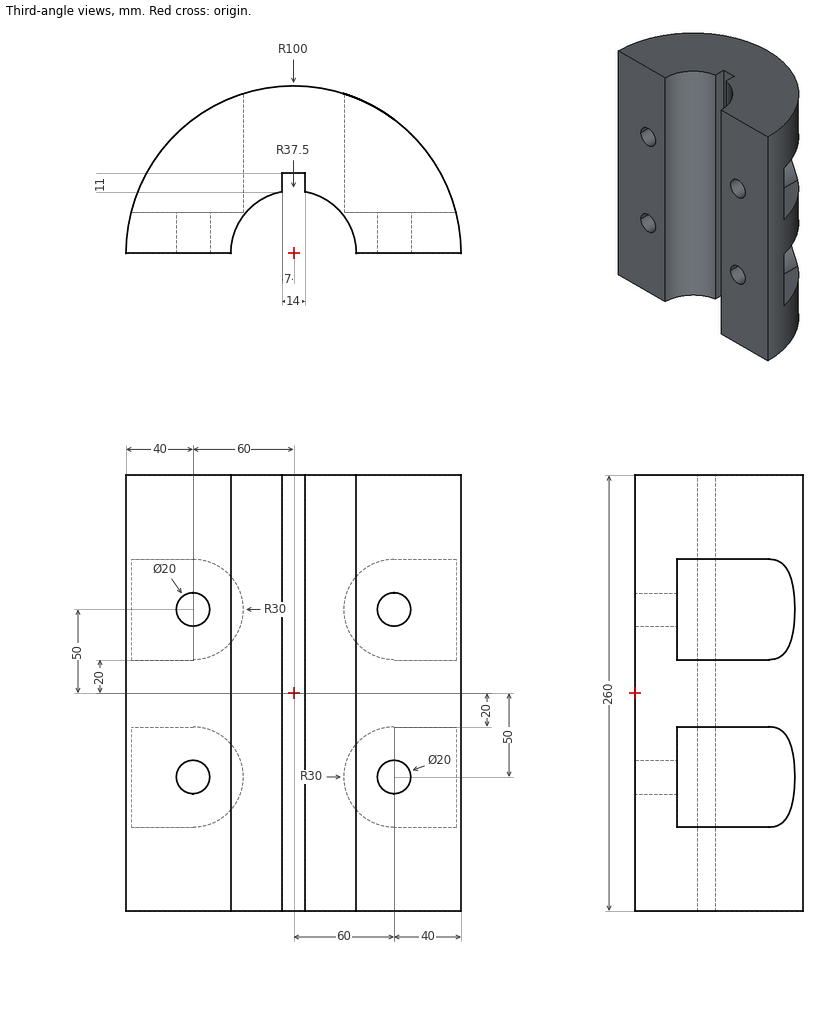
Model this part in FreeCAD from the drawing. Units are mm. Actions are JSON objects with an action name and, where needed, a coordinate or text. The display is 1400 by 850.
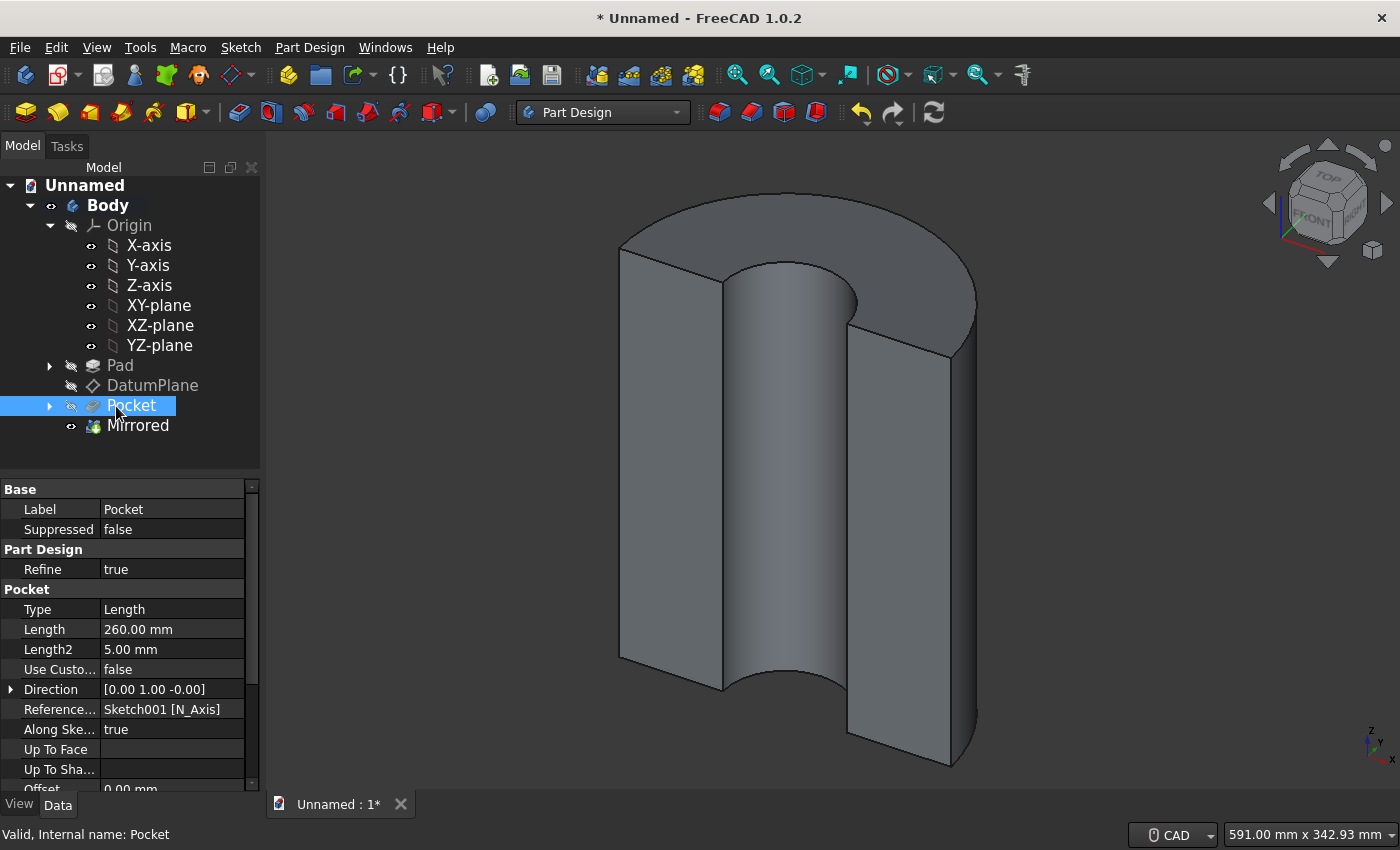
{"action": "left_click", "coordinate": [598, 76]}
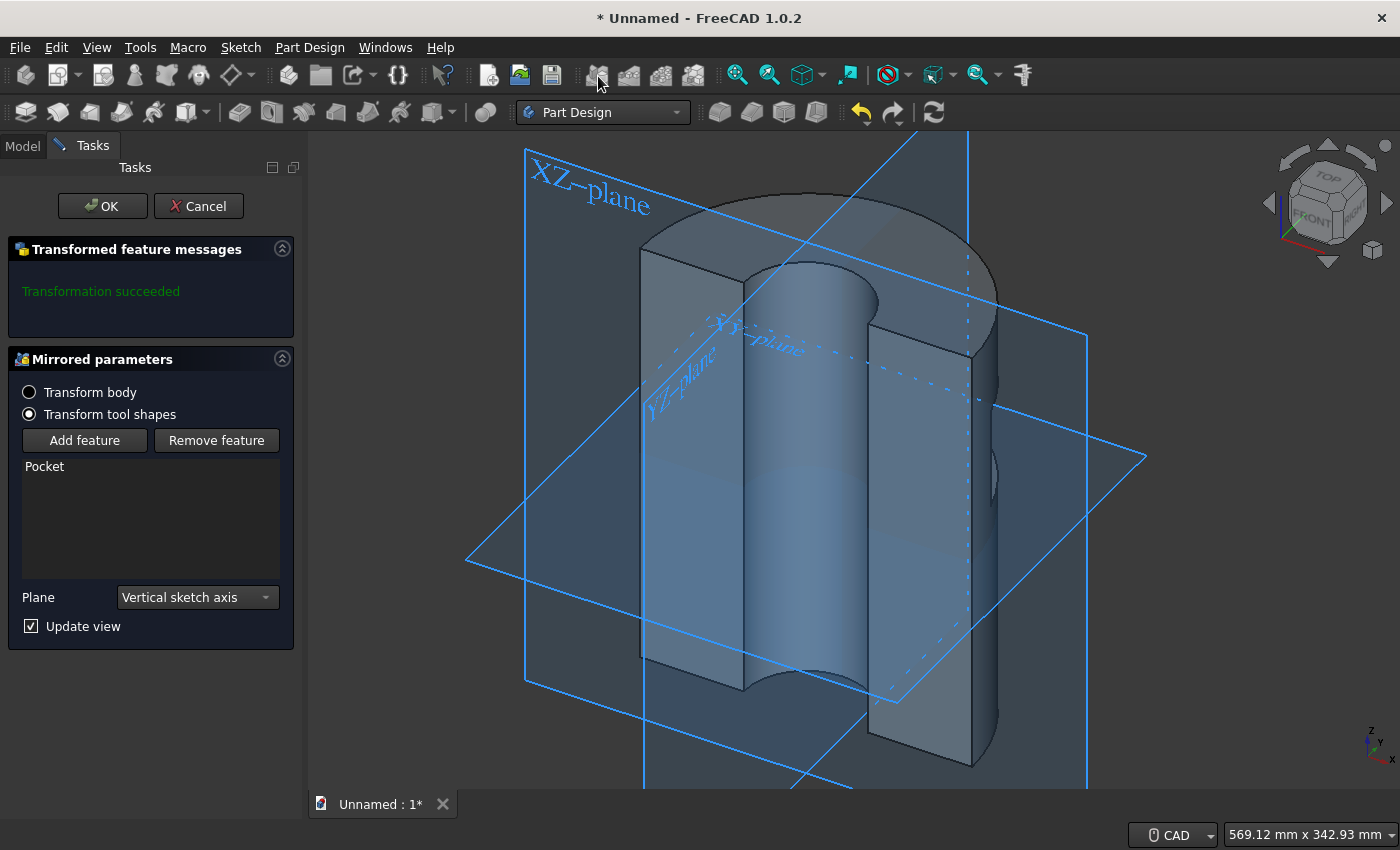
{"action": "left_click", "coordinate": [198, 598]}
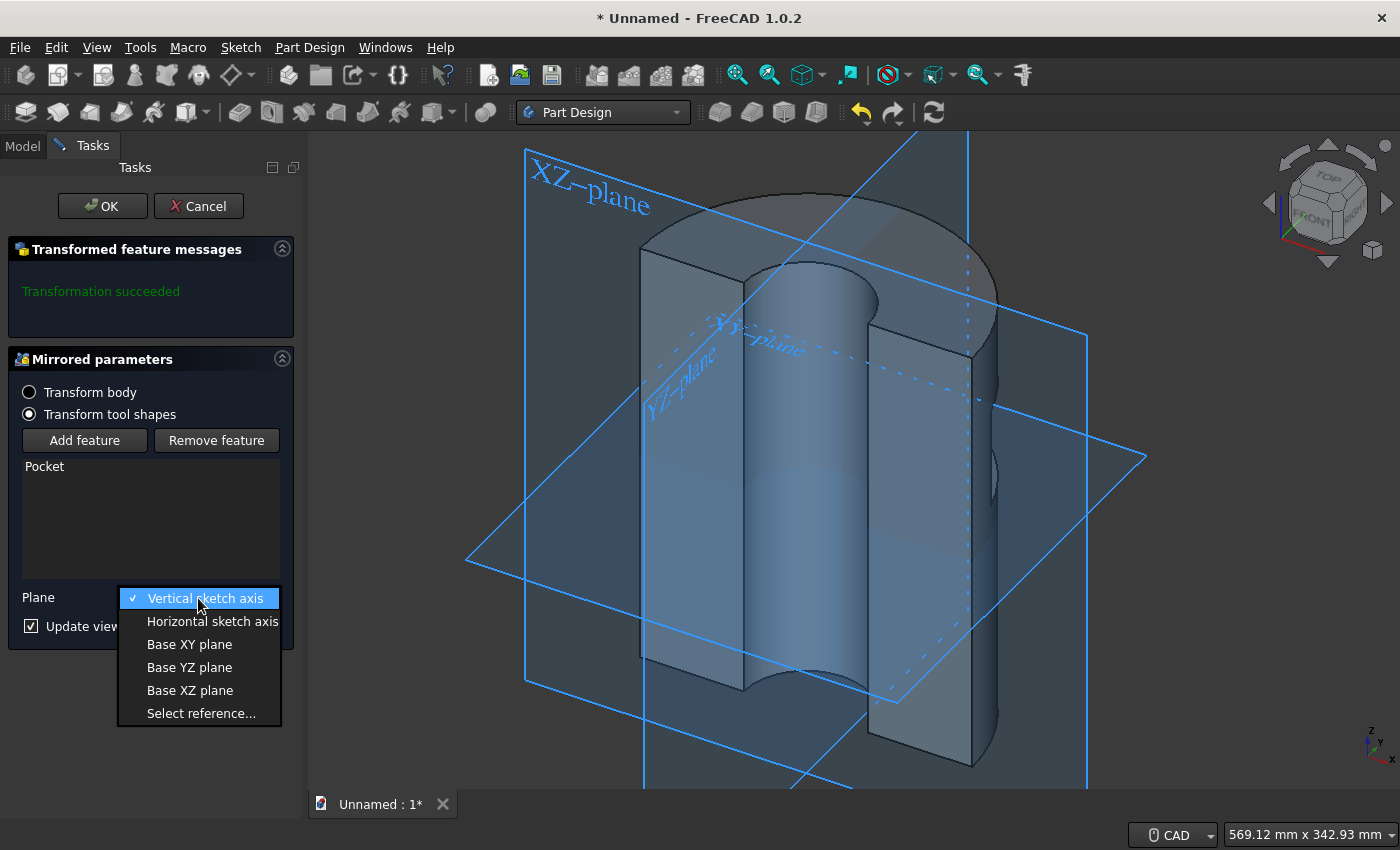
{"action": "left_click", "coordinate": [198, 668]}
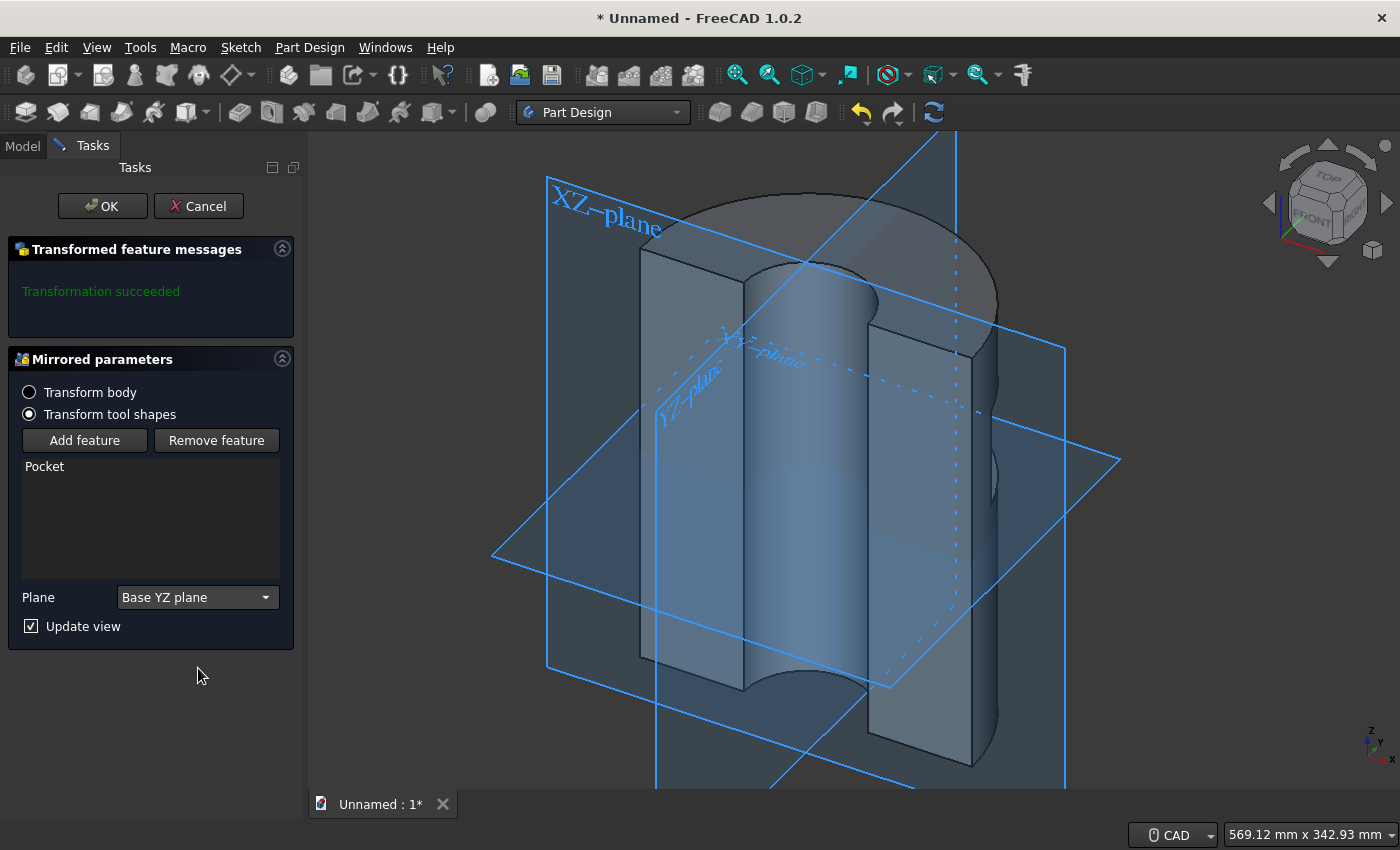
{"action": "left_click", "coordinate": [103, 206]}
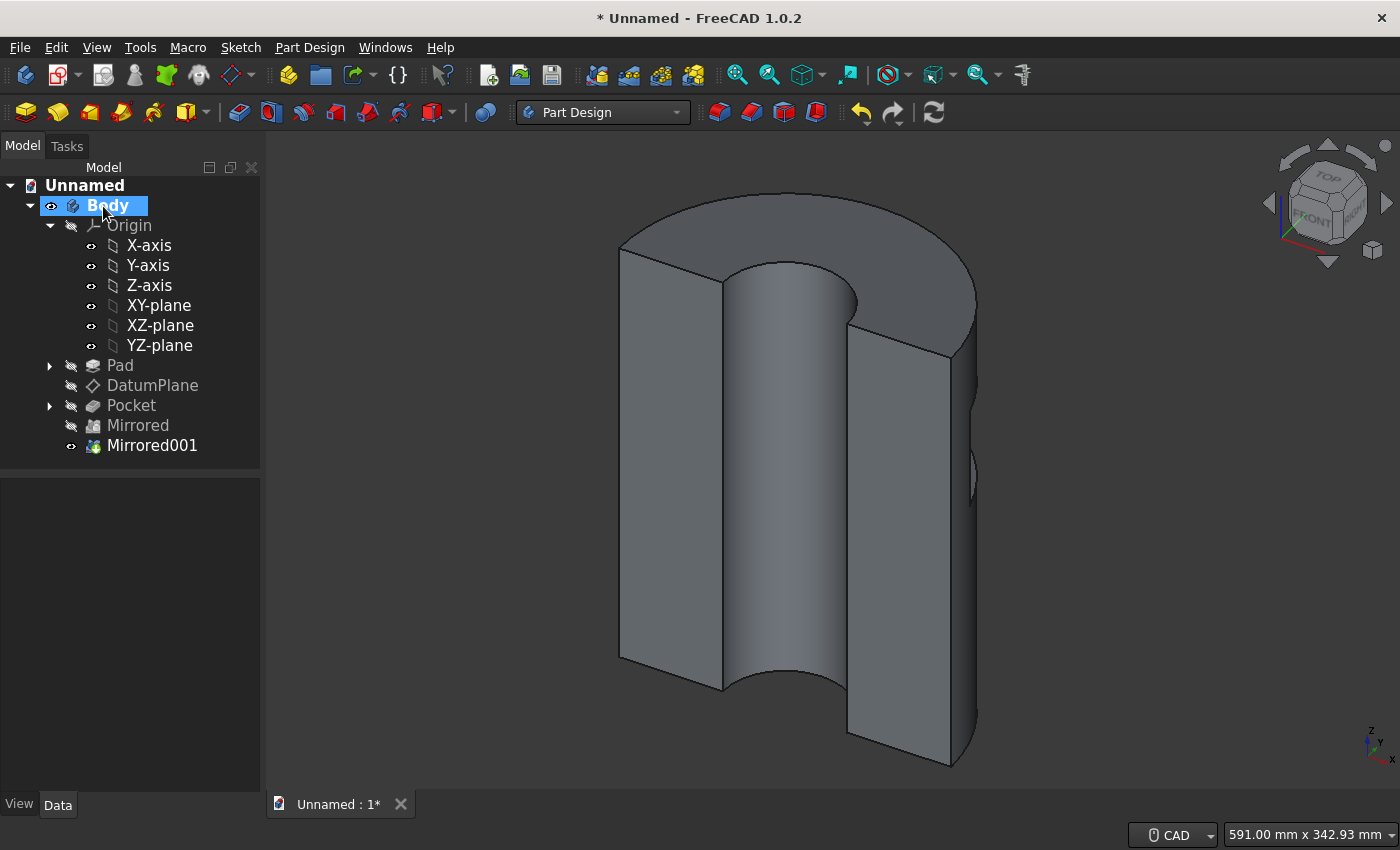
{"action": "key", "text": "4"}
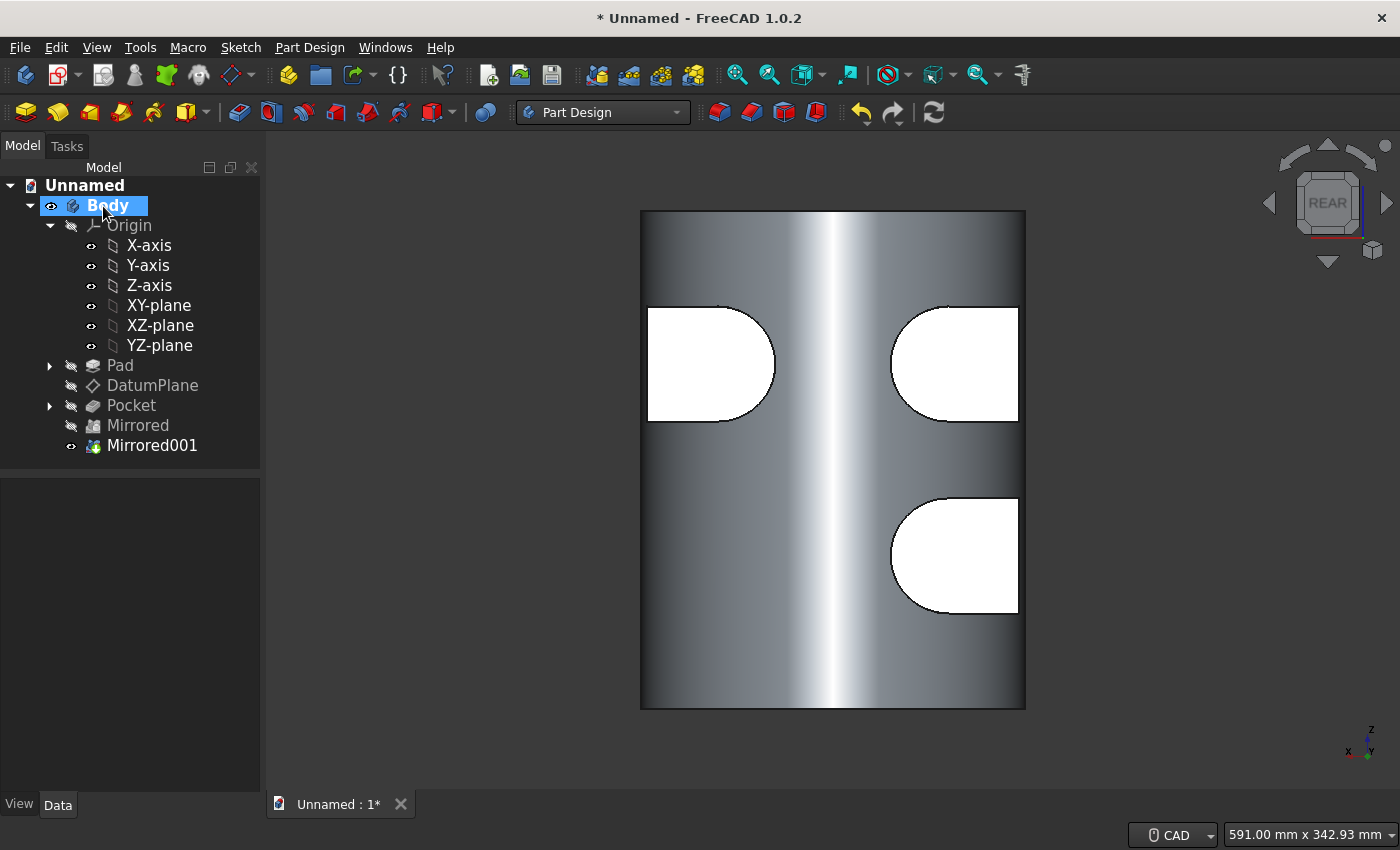
{"action": "left_click", "coordinate": [711, 363]}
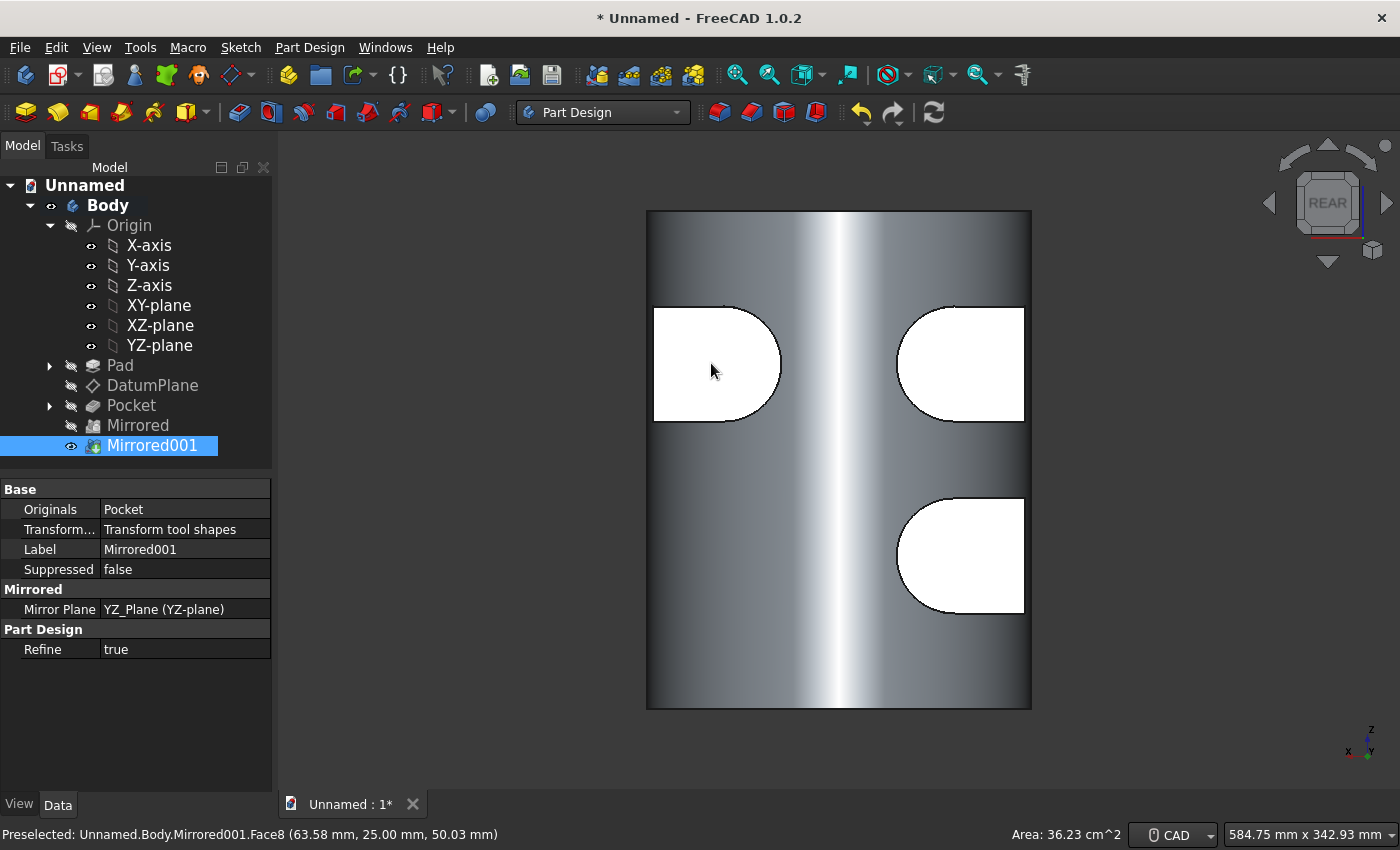
{"action": "left_click", "coordinate": [58, 76]}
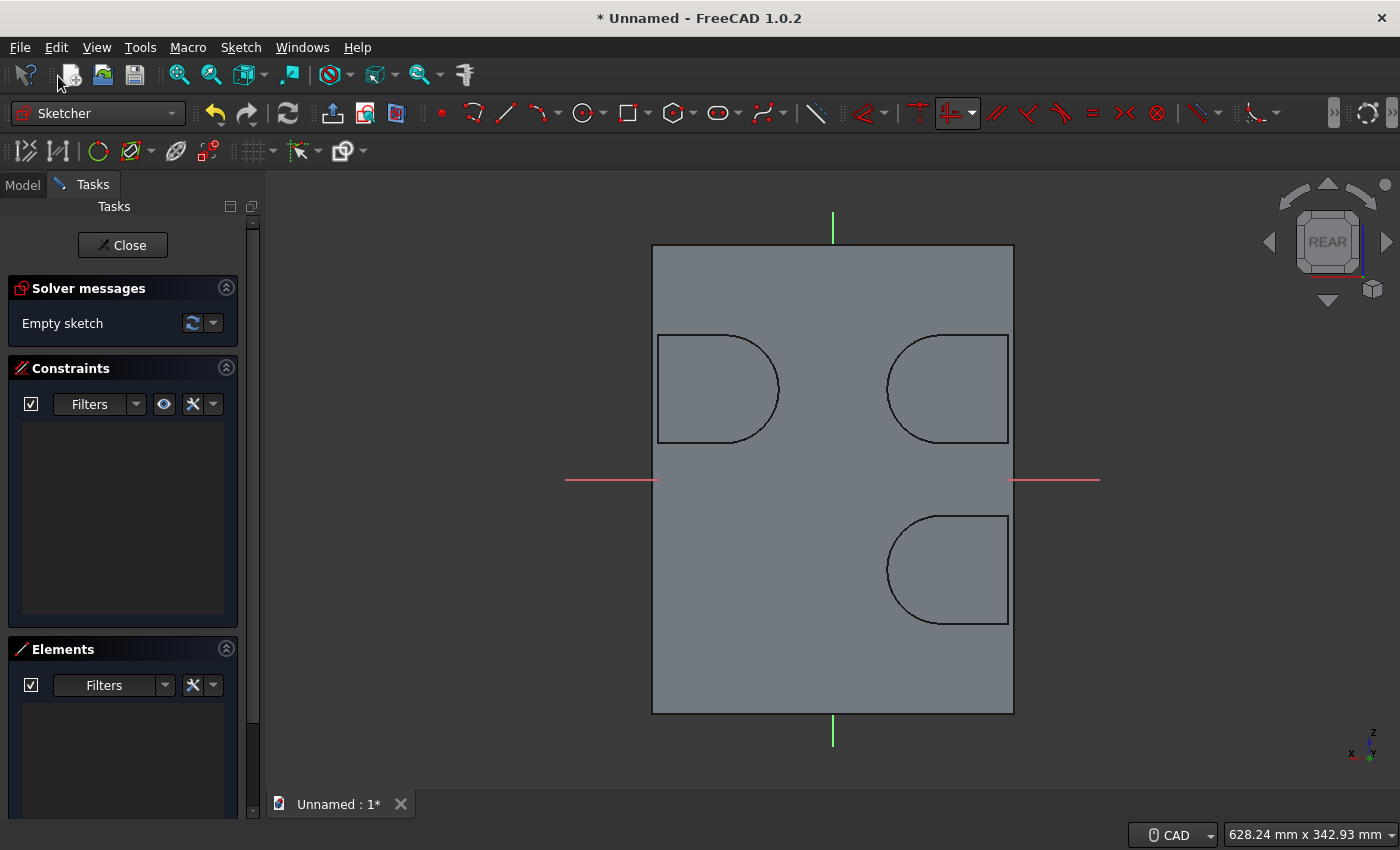
{"action": "left_click", "coordinate": [398, 114]}